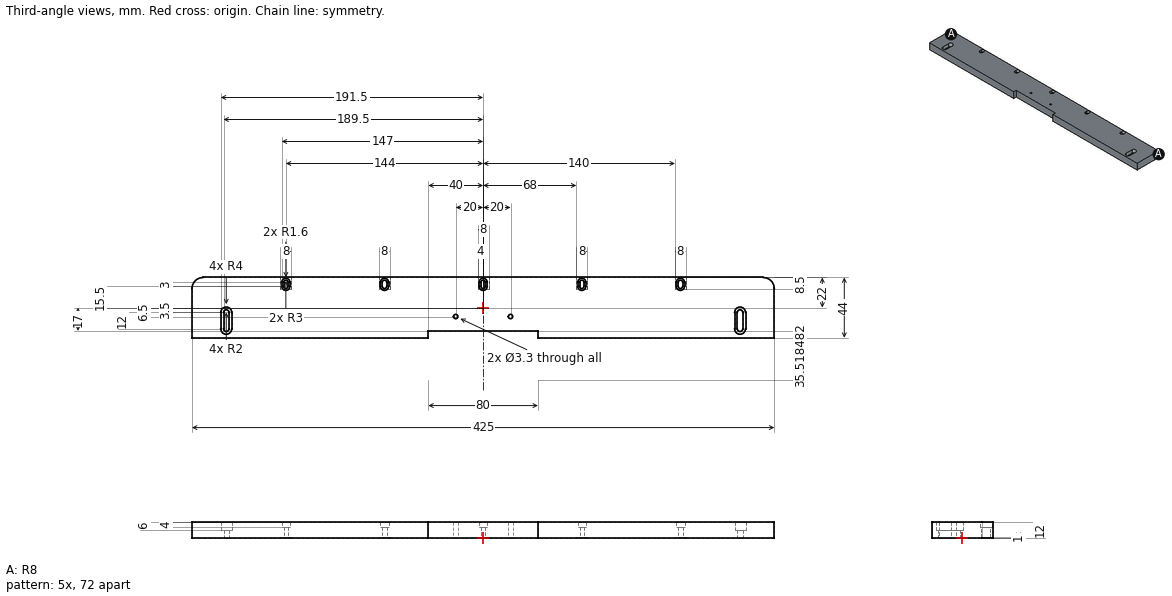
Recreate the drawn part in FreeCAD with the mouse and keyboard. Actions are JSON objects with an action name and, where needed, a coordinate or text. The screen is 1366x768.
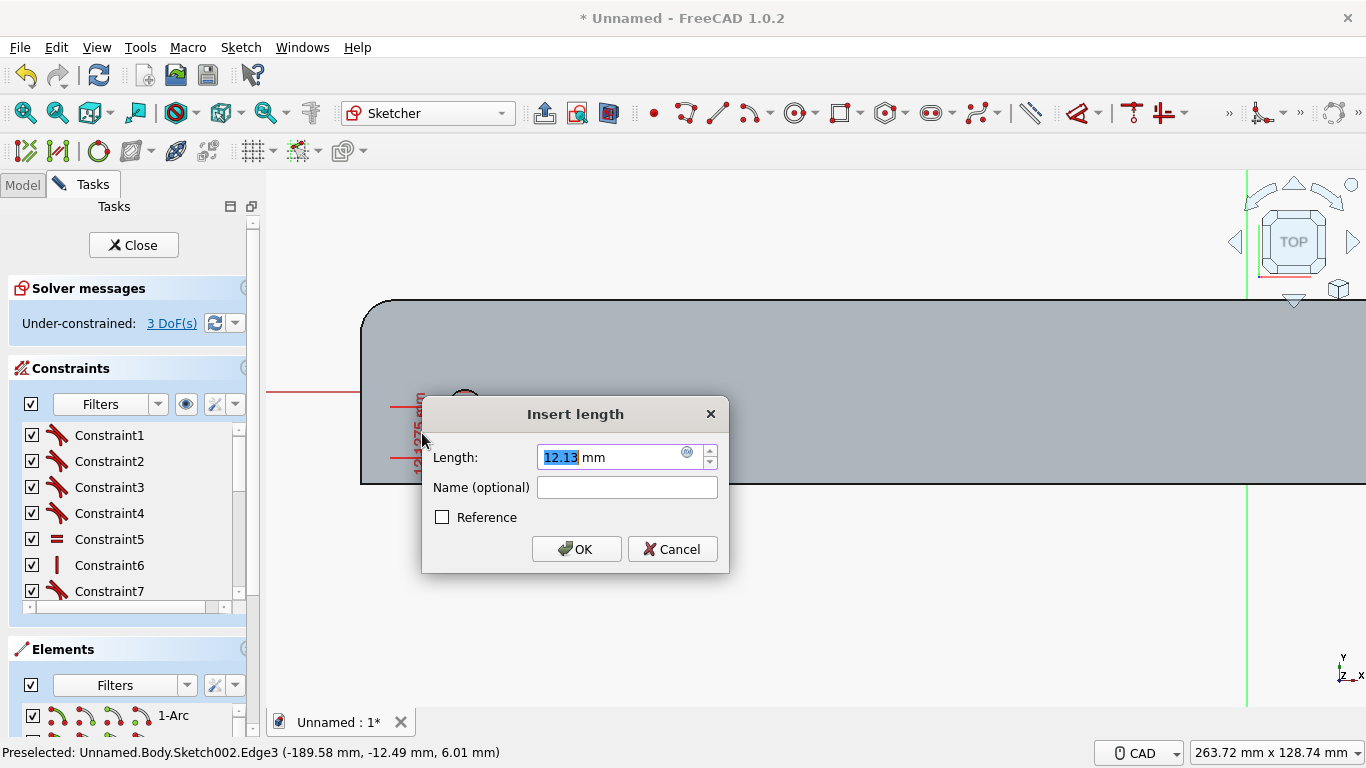
{"action": "type", "text": "12"}
{"action": "key", "text": "Return"}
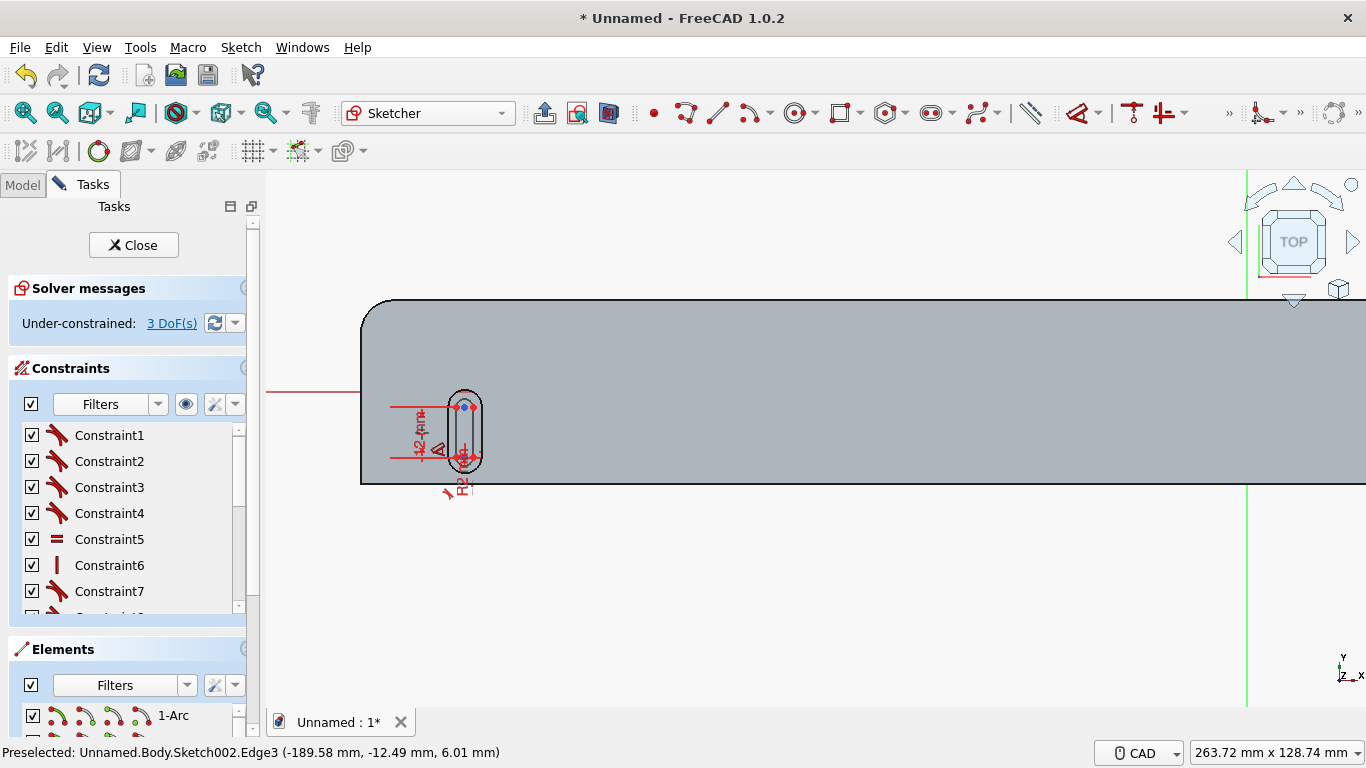
{"action": "scroll", "coordinate": [457, 444], "scroll_direction": "down", "scroll_amount": 5}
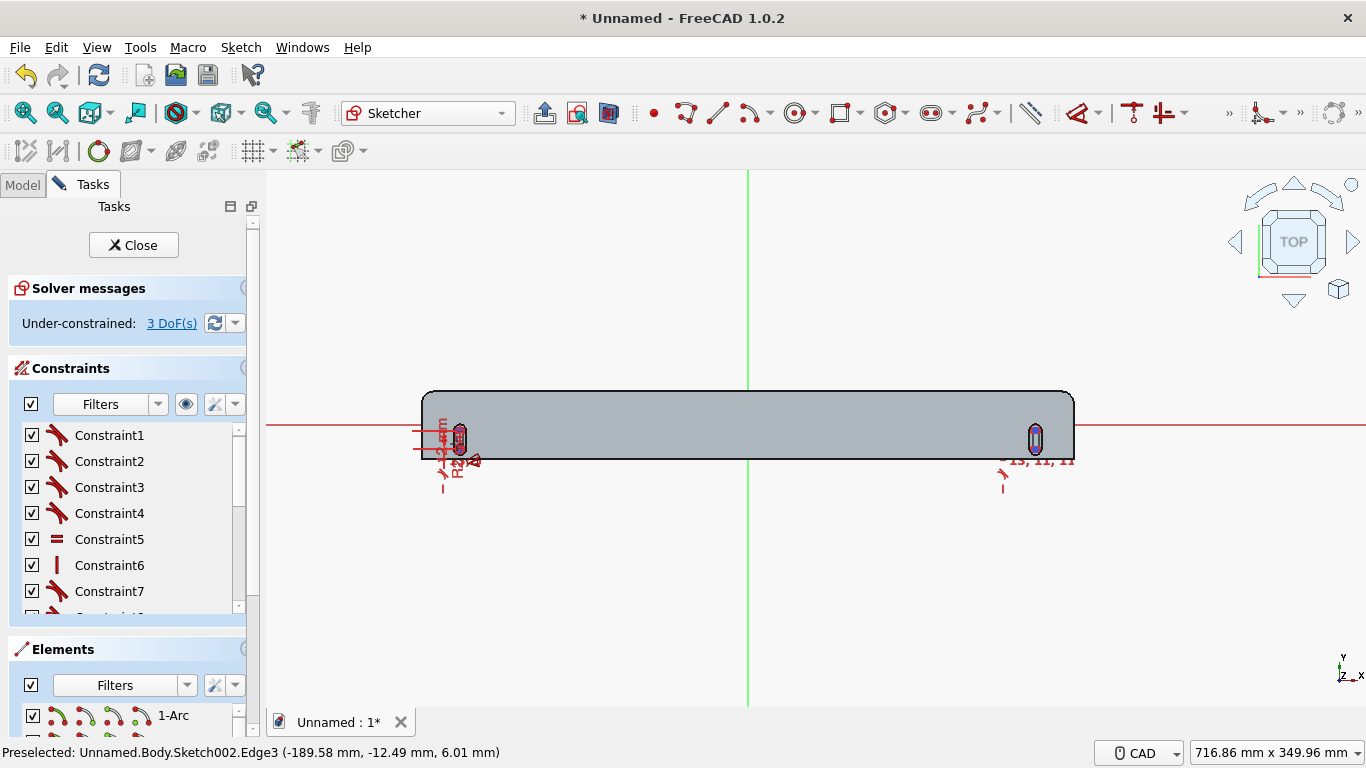
{"action": "scroll", "coordinate": [1033, 444], "scroll_direction": "up", "scroll_amount": 5}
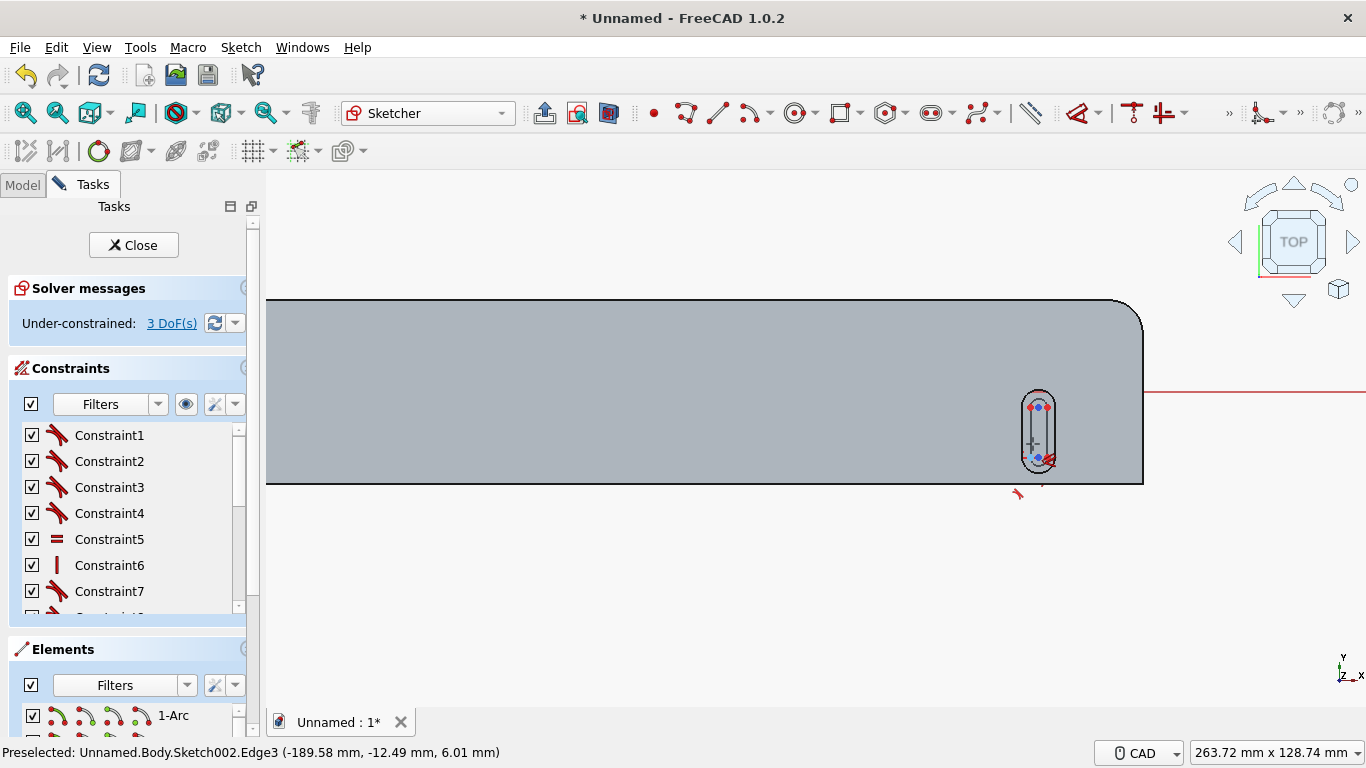
{"action": "left_click", "coordinate": [1031, 442]}
{"action": "left_click", "coordinate": [1065, 432]}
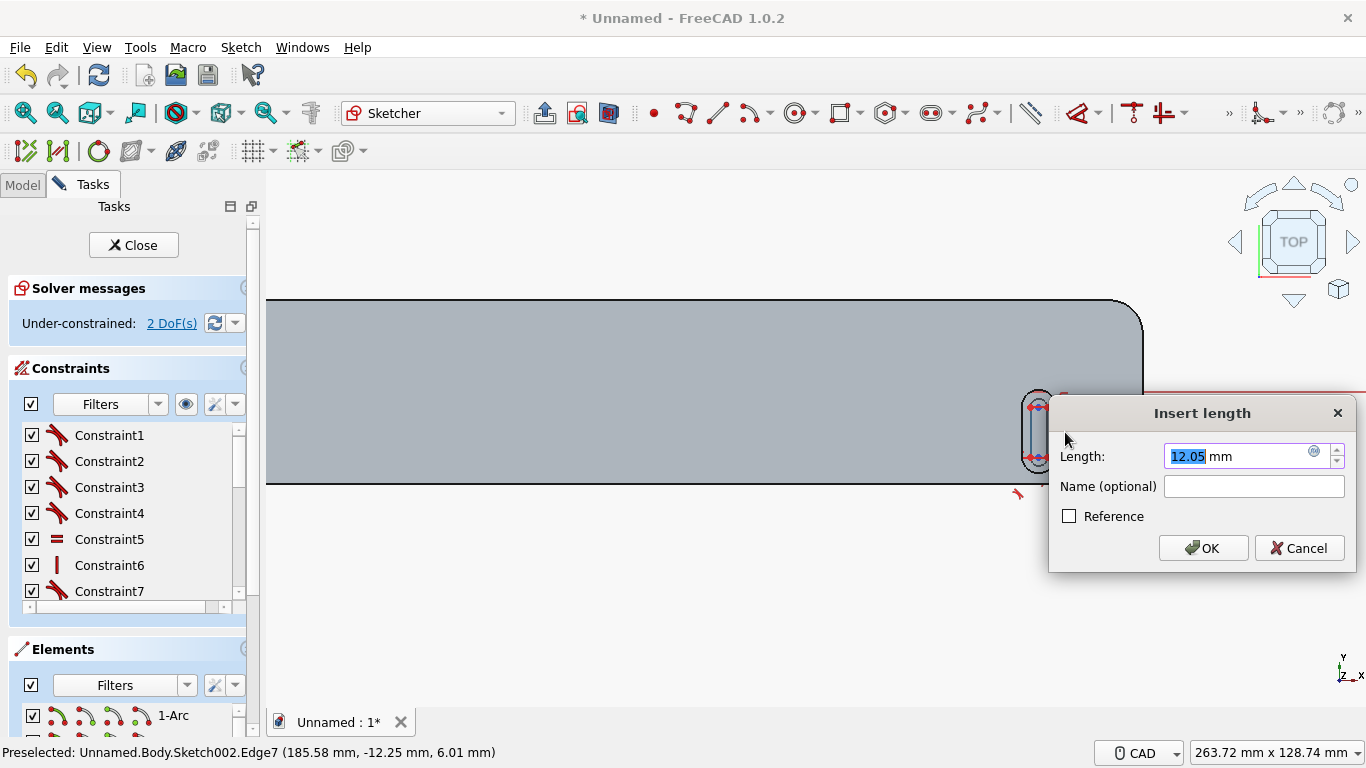
{"action": "type", "text": "12"}
{"action": "key", "text": "Return"}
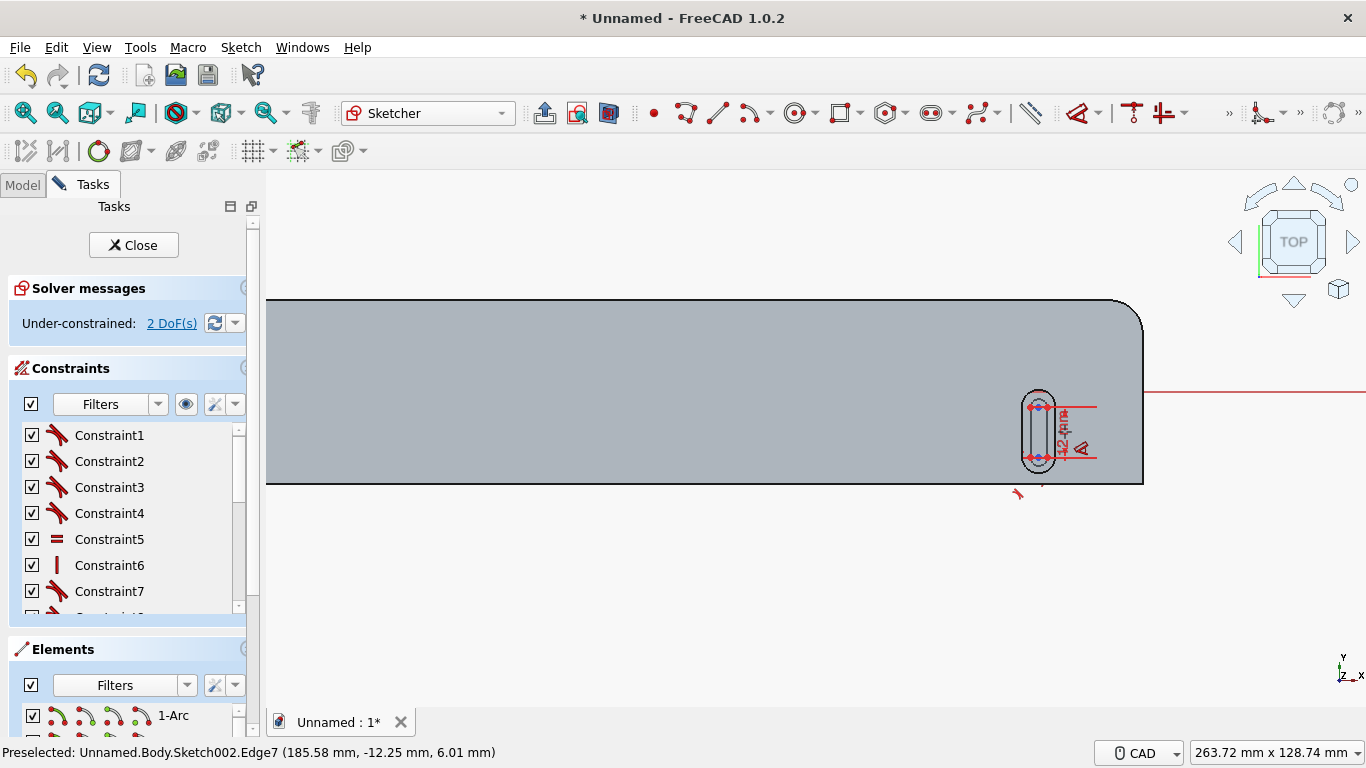
{"action": "scroll", "coordinate": [1033, 444], "scroll_direction": "down", "scroll_amount": 5}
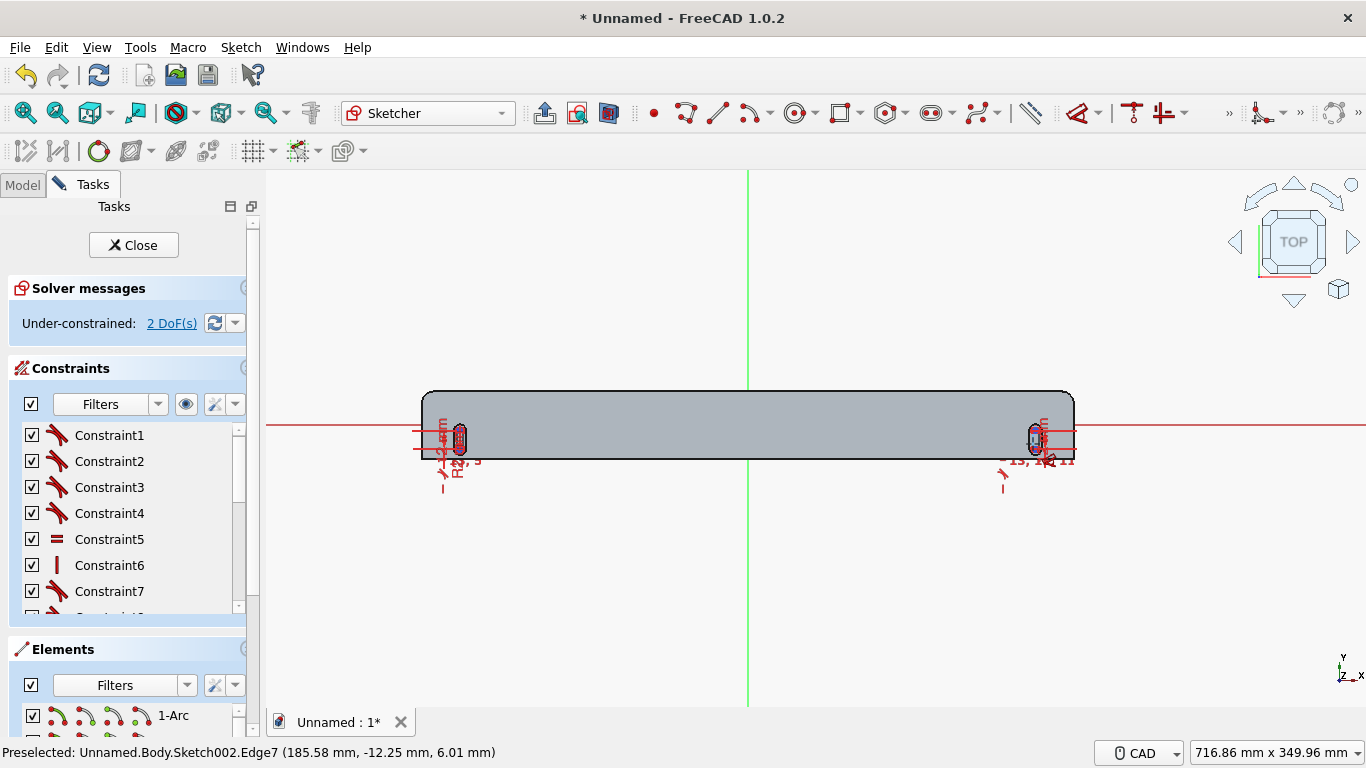
{"action": "scroll", "coordinate": [463, 431], "scroll_direction": "up", "scroll_amount": 11}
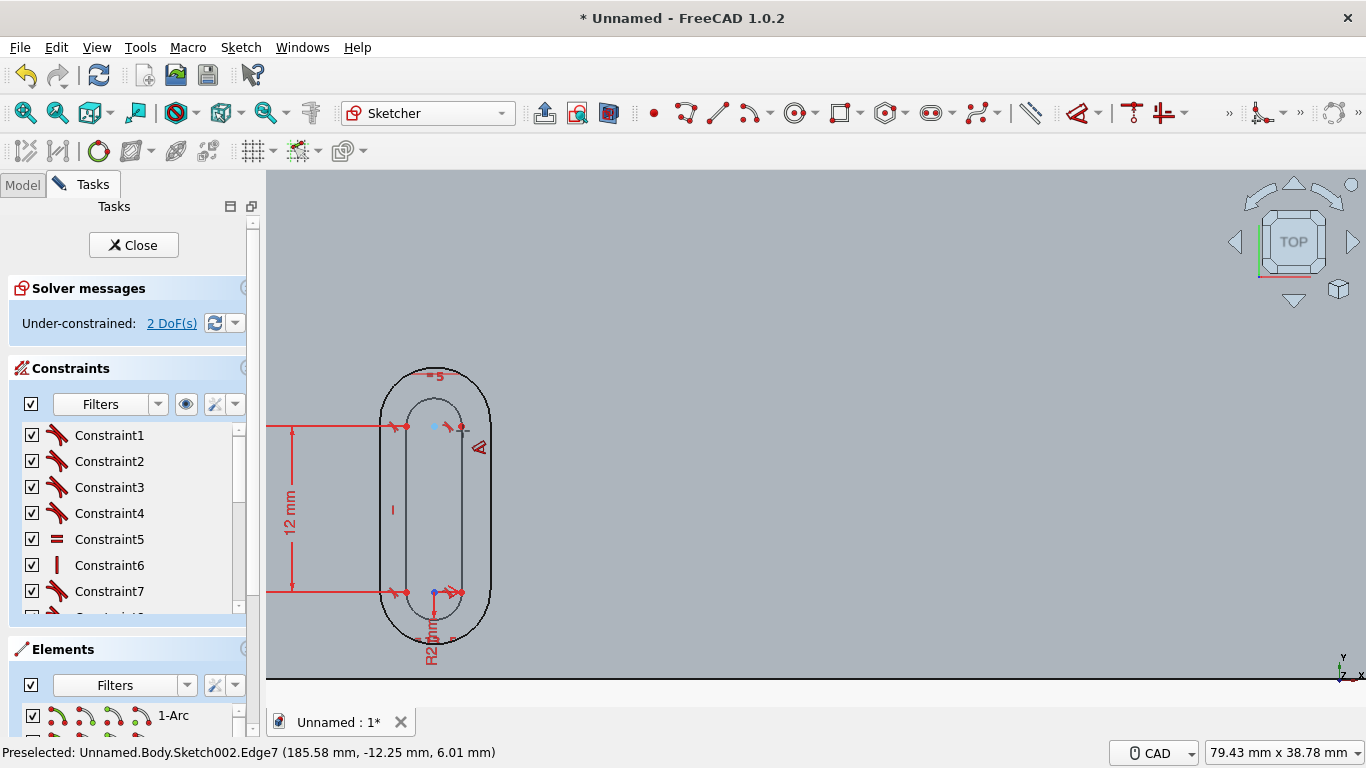
{"action": "left_click", "coordinate": [462, 426]}
{"action": "left_click", "coordinate": [428, 418]}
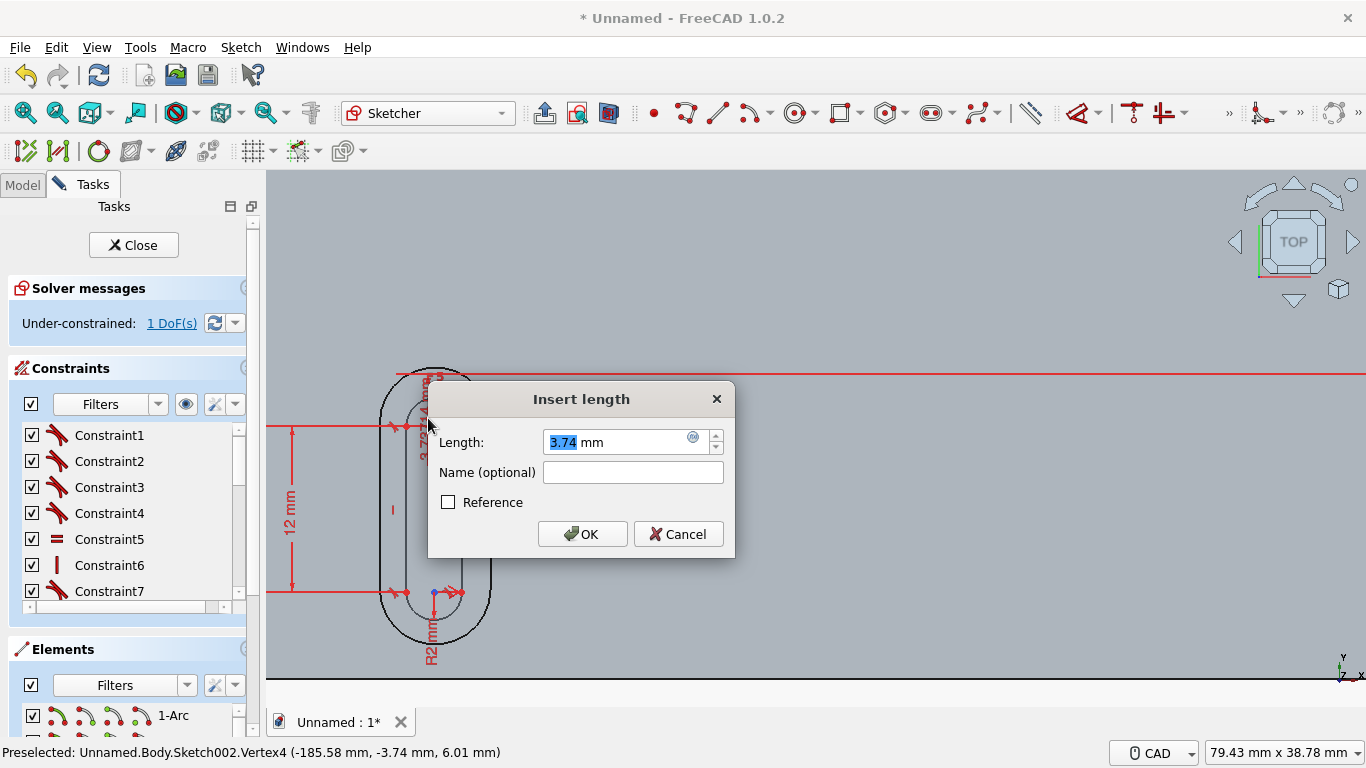
{"action": "type", "text": "3.5"}
{"action": "key", "text": "Return"}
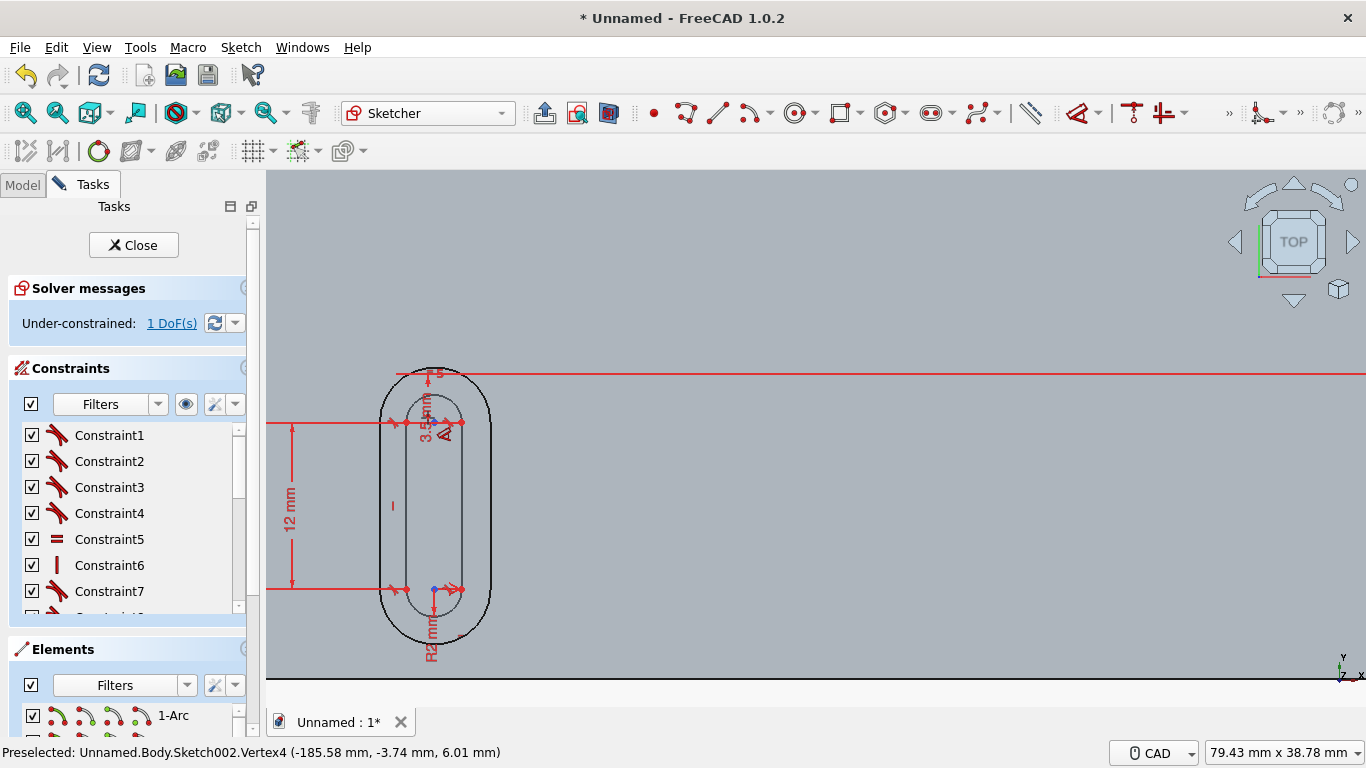
{"action": "left_click", "coordinate": [406, 589]}
{"action": "left_click", "coordinate": [804, 340]}